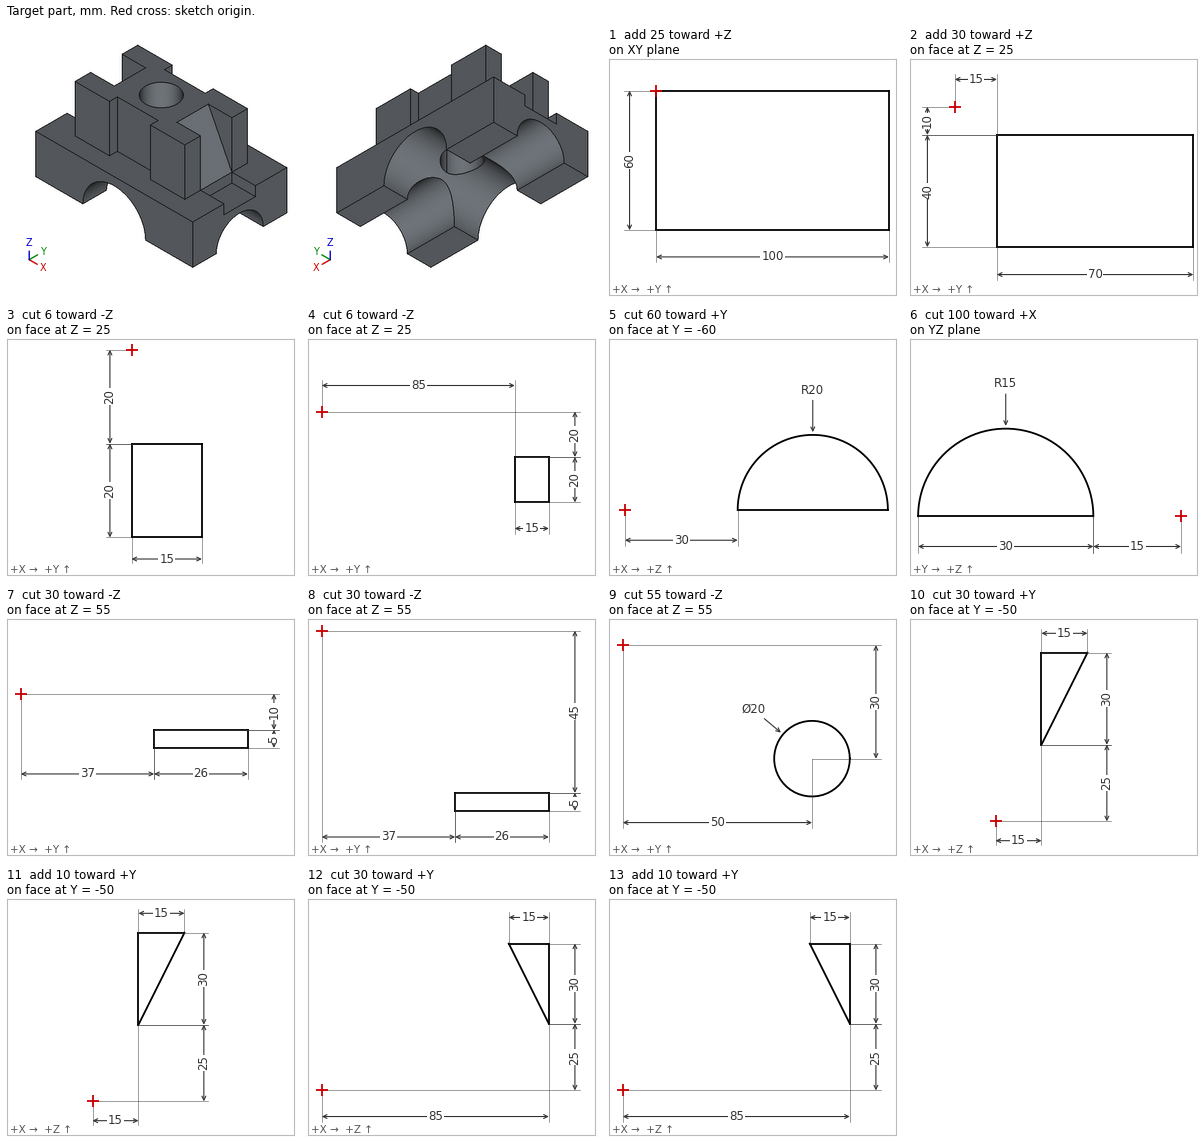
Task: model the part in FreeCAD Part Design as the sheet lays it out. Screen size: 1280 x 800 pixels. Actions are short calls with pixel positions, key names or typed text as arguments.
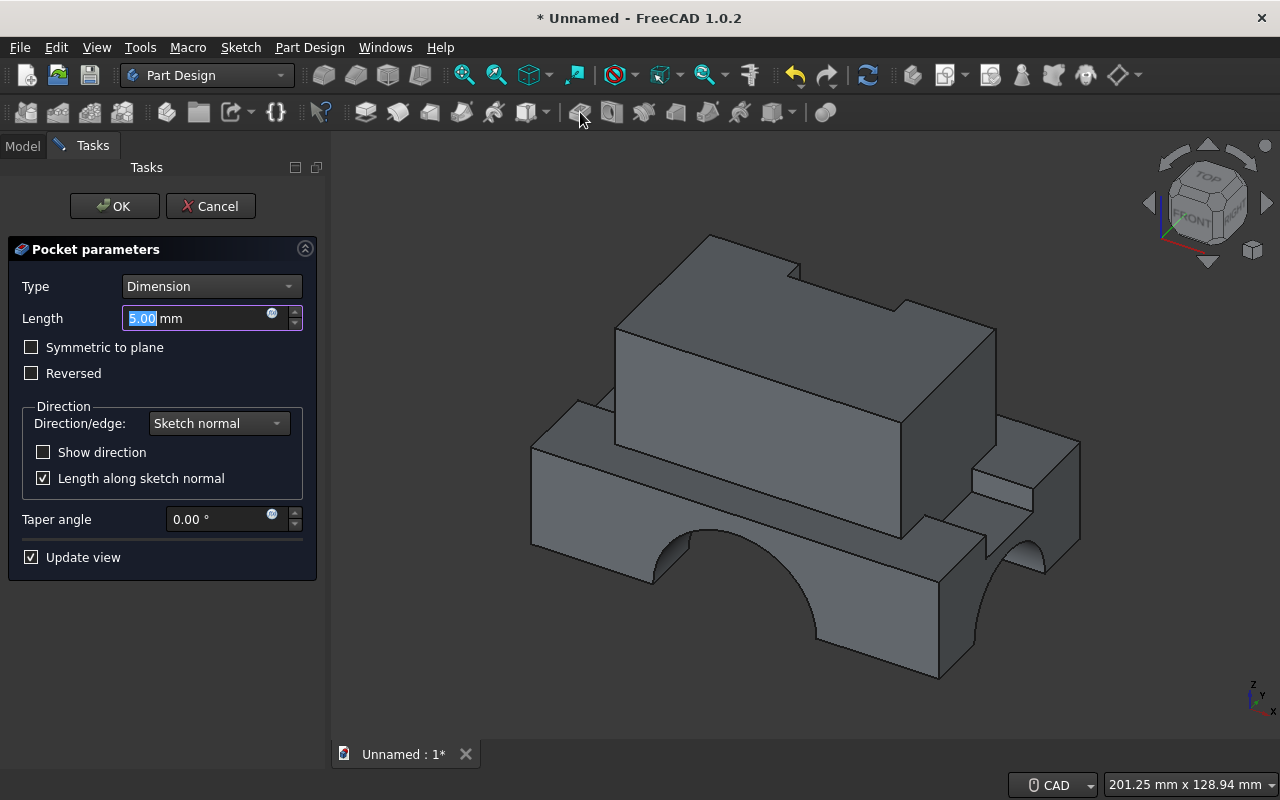
text(30)
key(Tab)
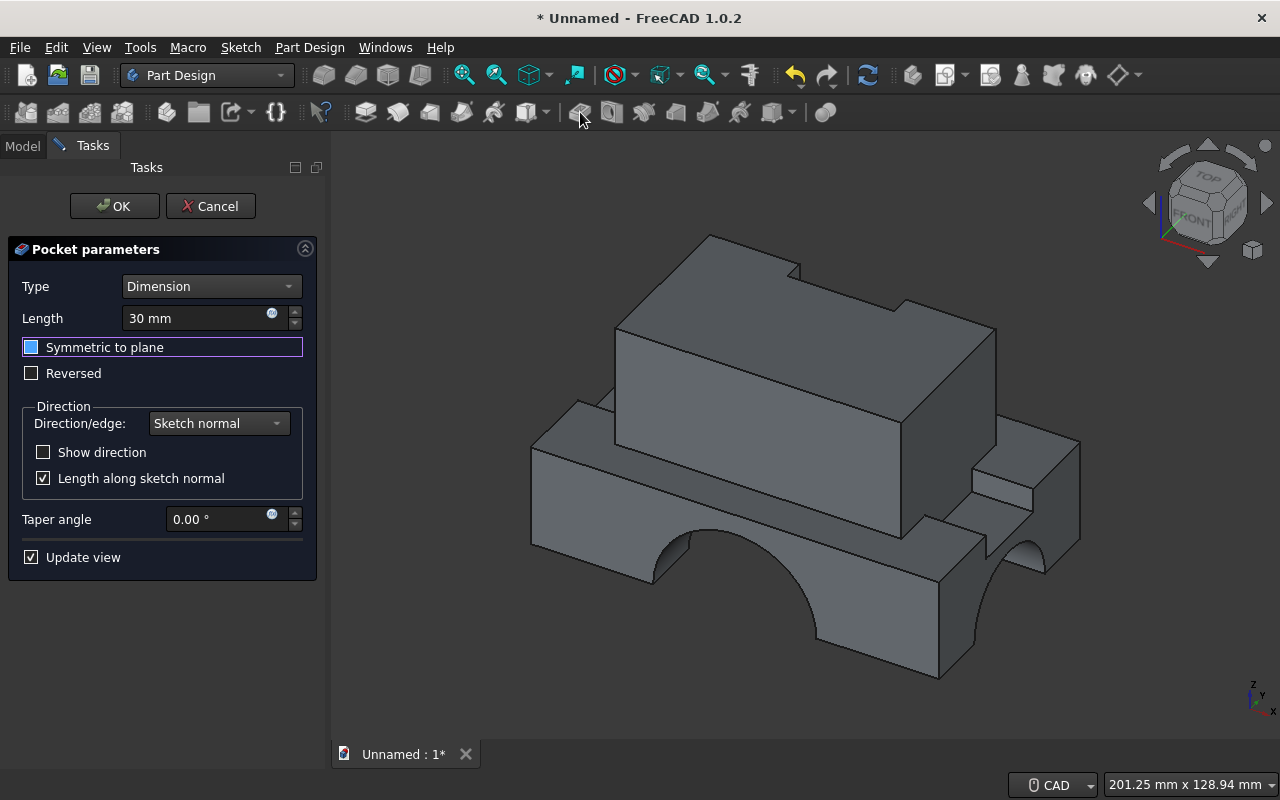
click(115, 206)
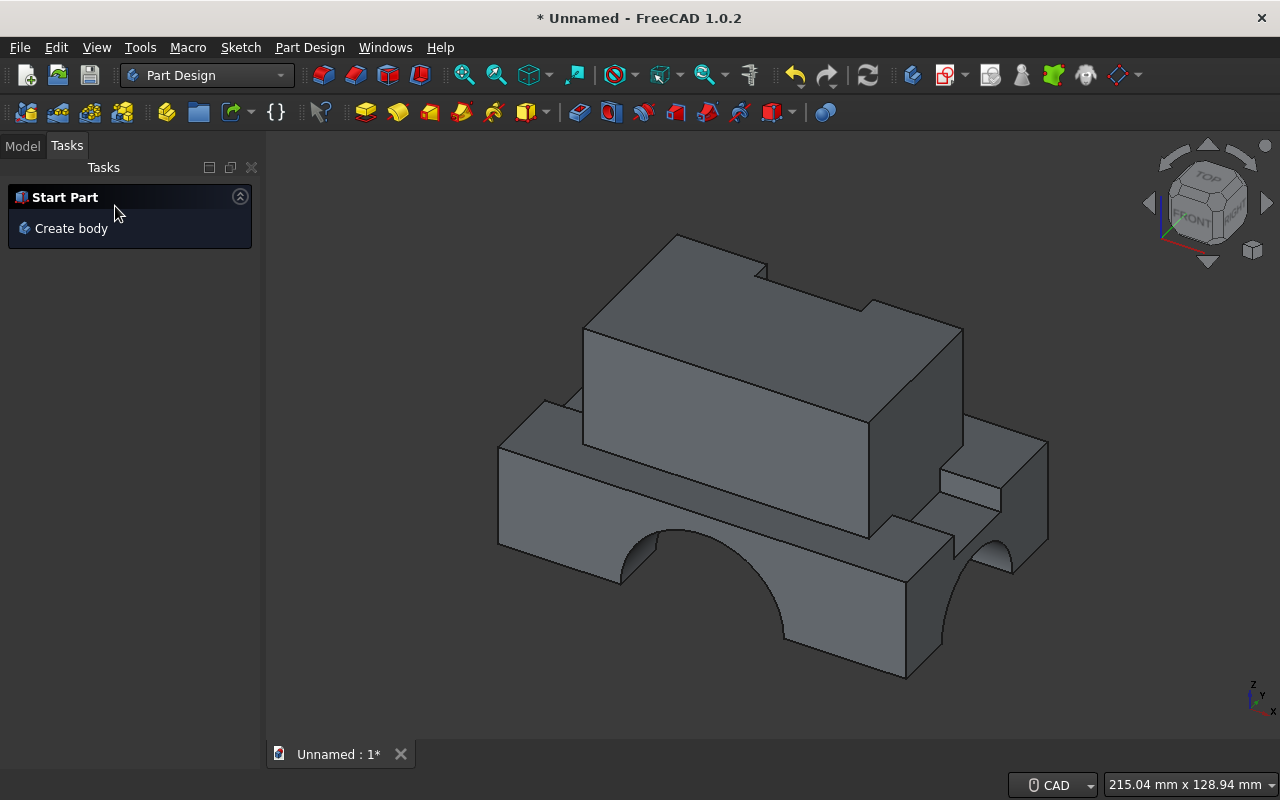
click(855, 355)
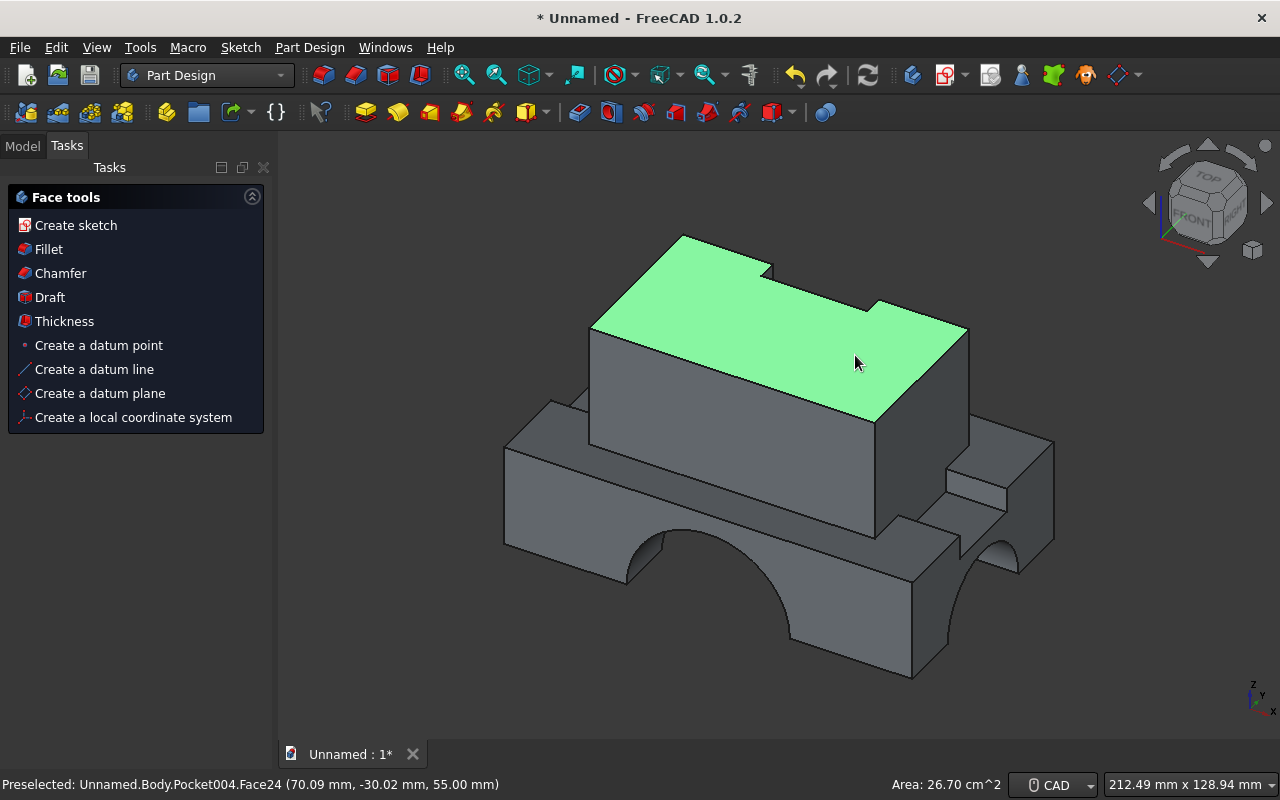
click(946, 76)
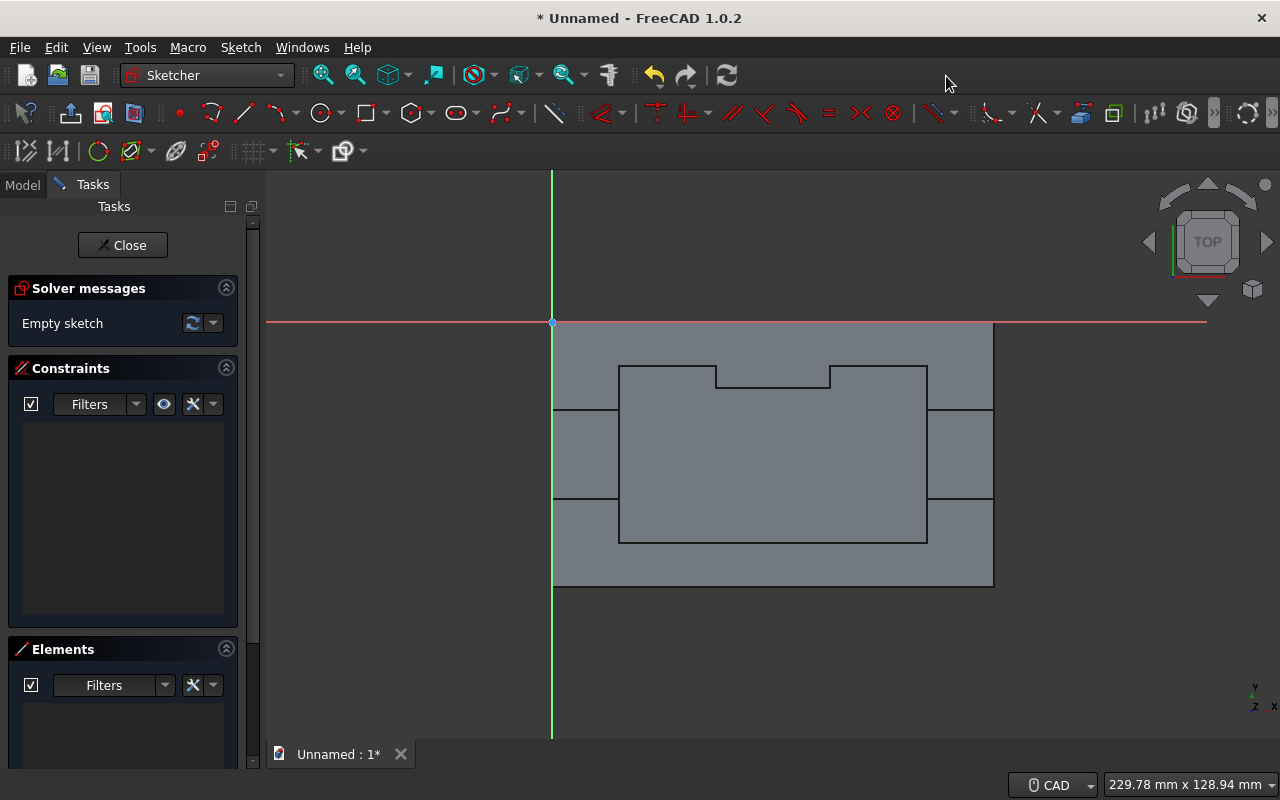
scroll(665, 388, up, 2)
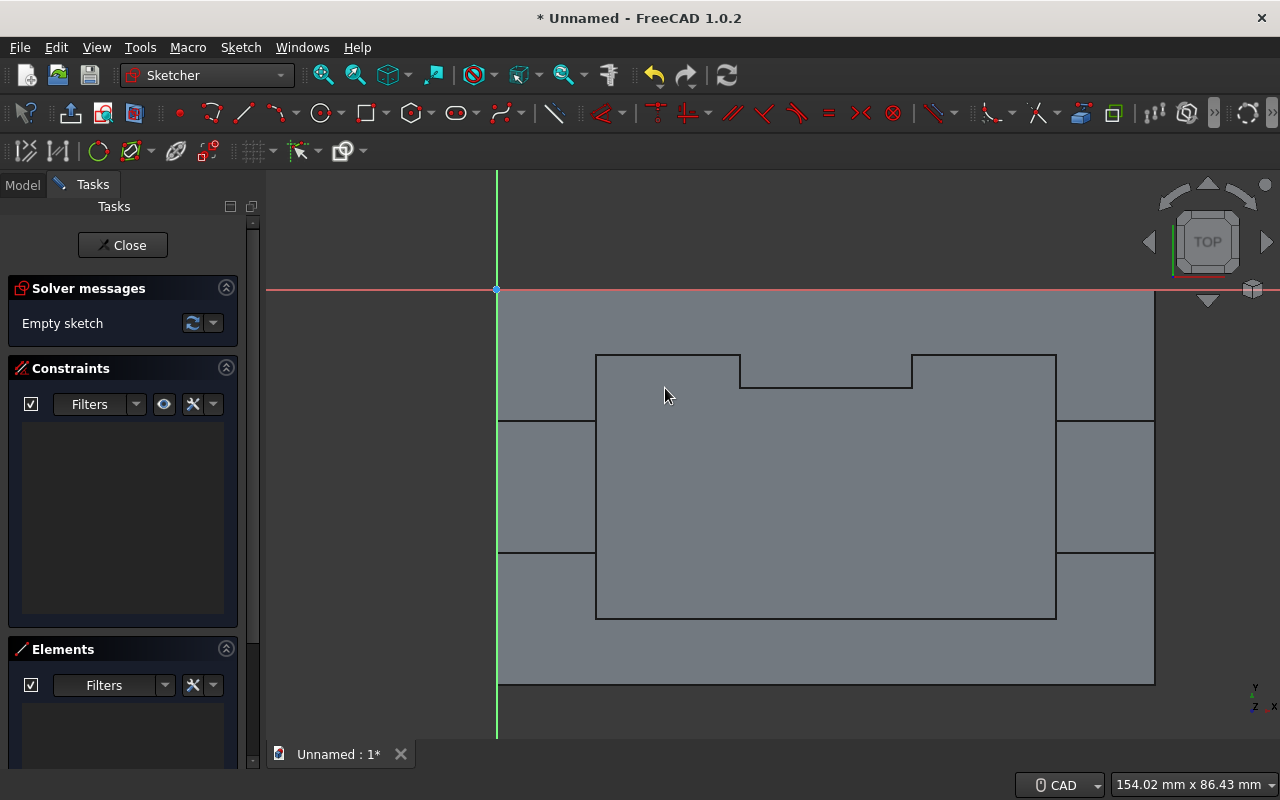
click(366, 114)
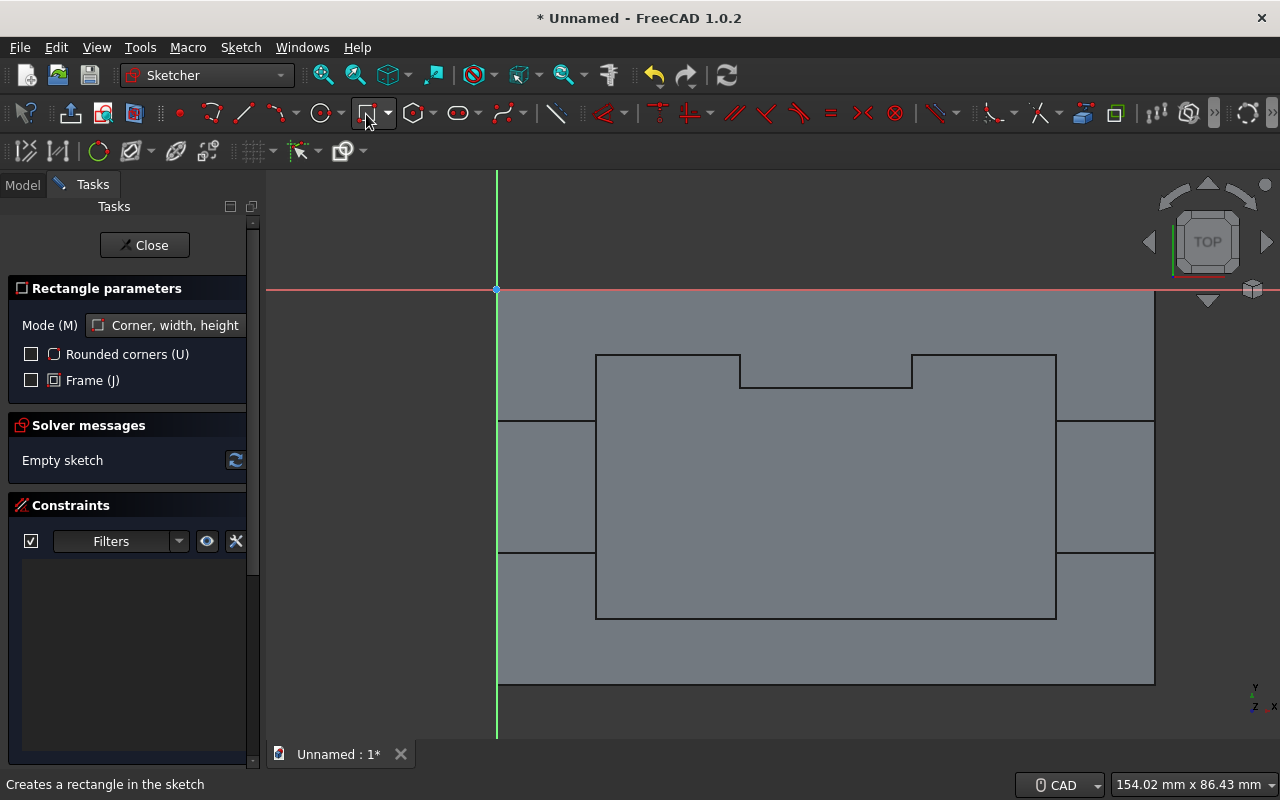
click(740, 586)
click(912, 619)
key(Escape)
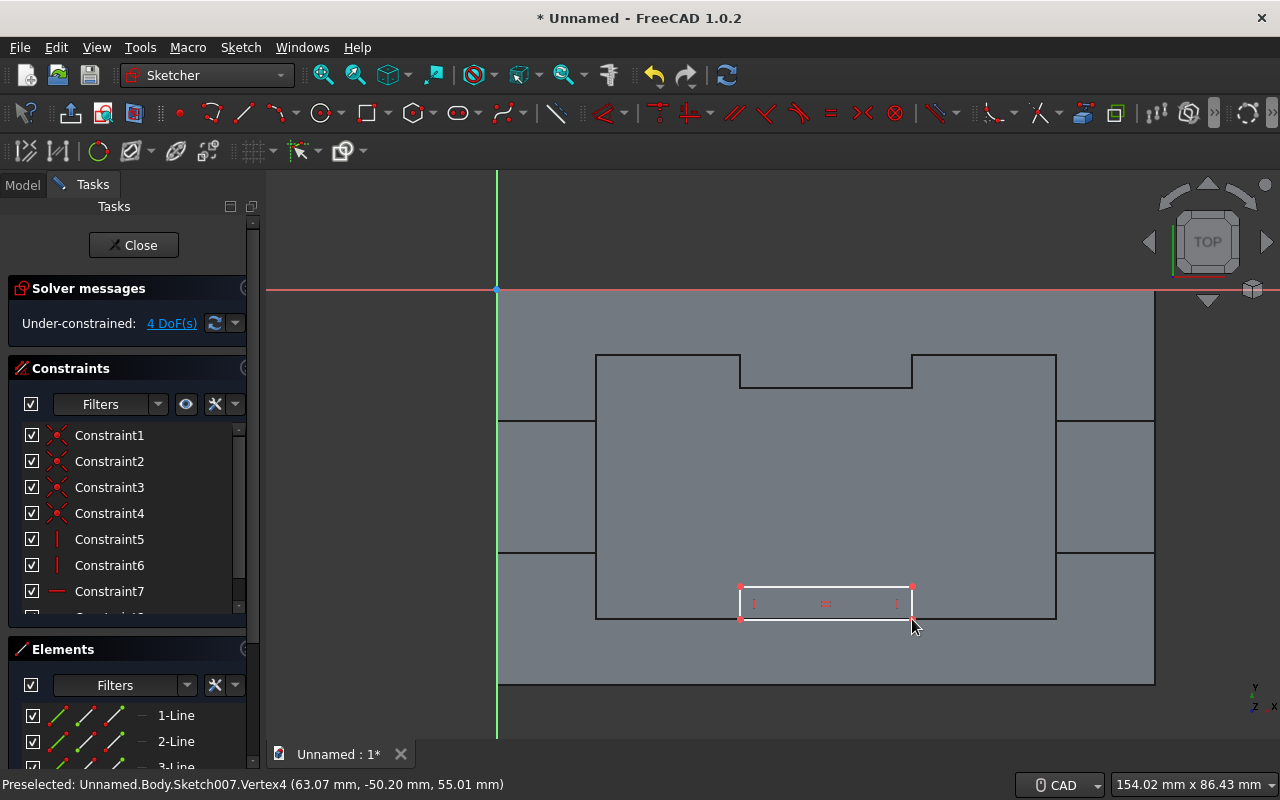
key(d)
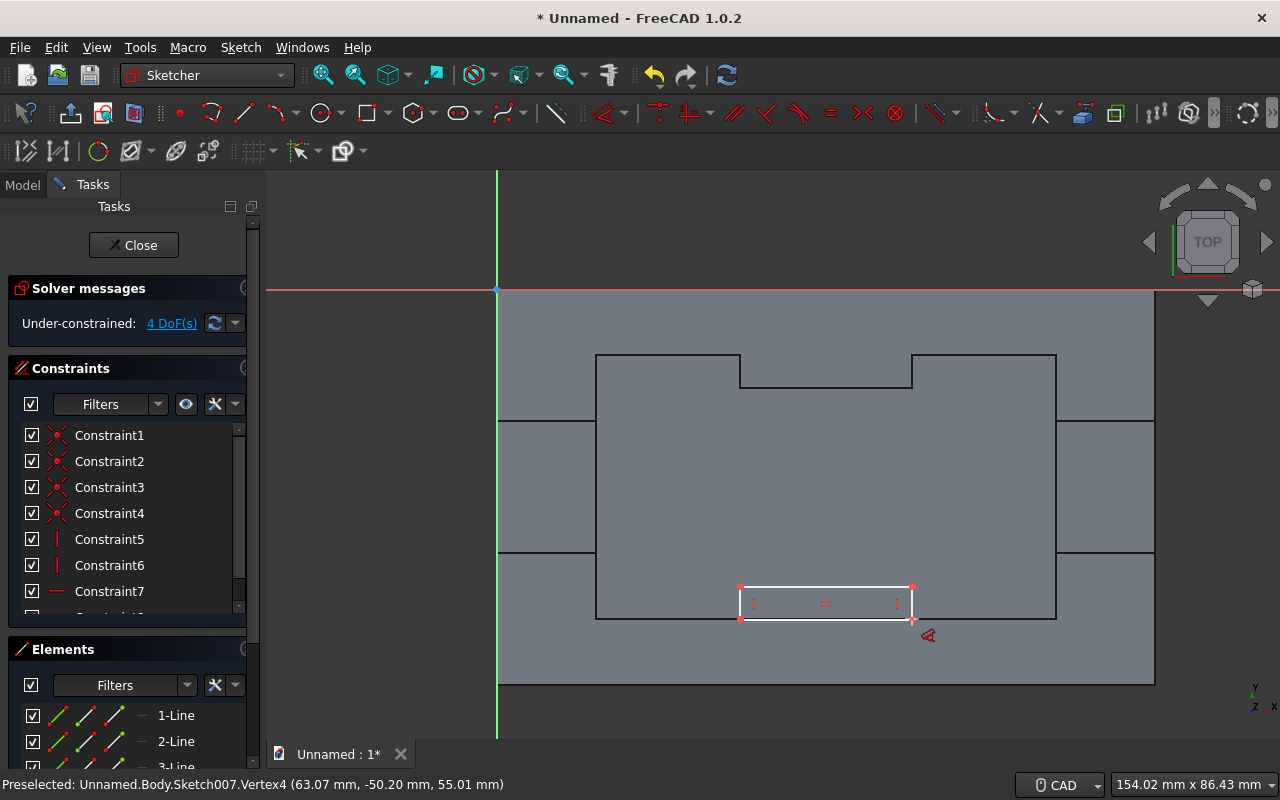
scroll(740, 597, up, 2)